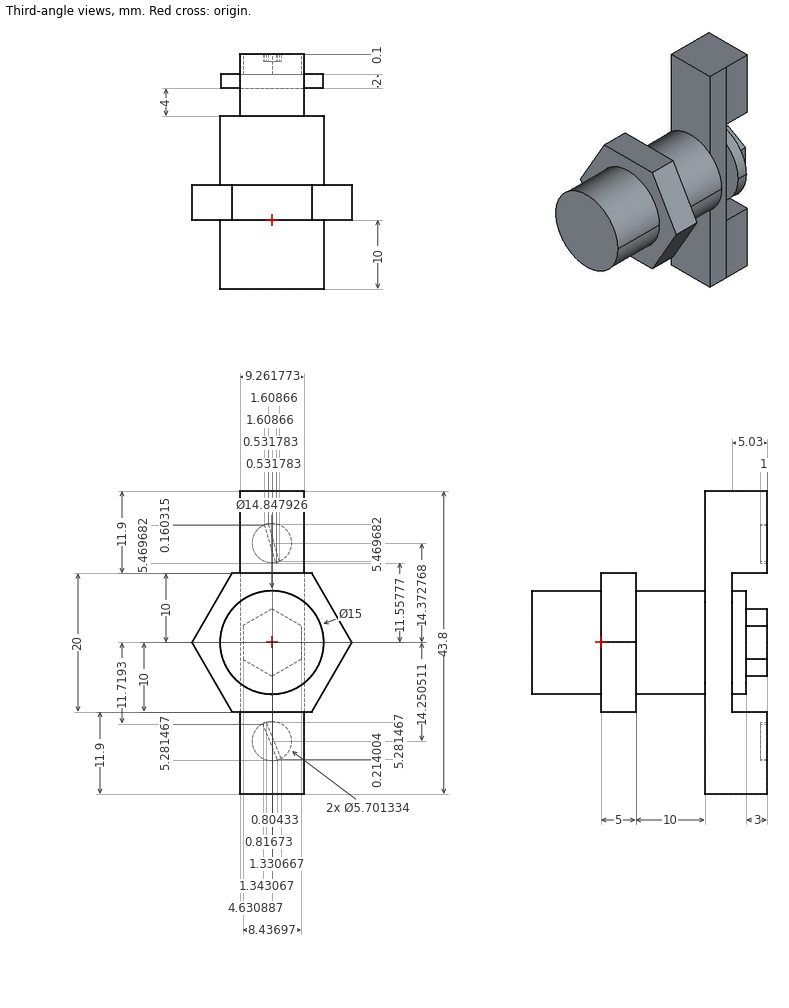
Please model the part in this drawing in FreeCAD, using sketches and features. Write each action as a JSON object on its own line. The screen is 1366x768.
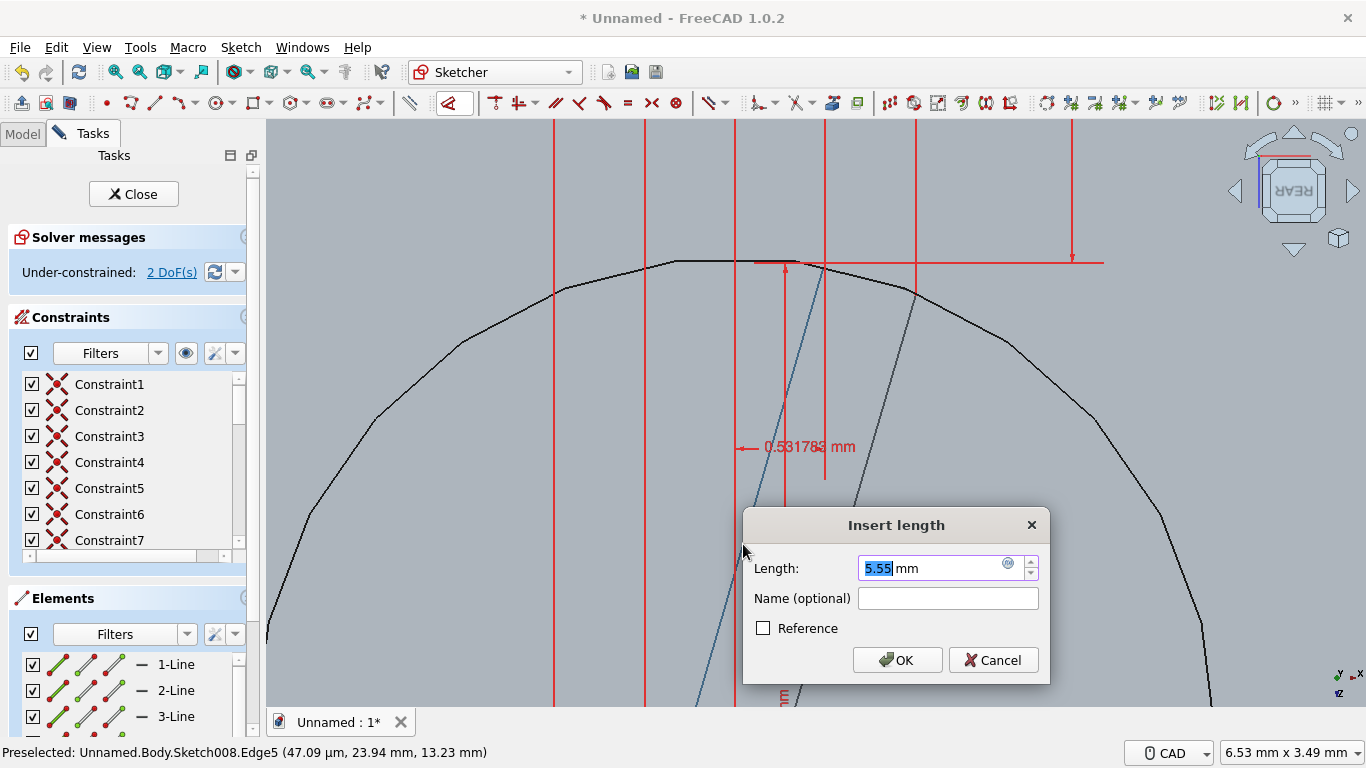
{"action": "type", "text": "5.469682"}
{"action": "key", "text": "Return"}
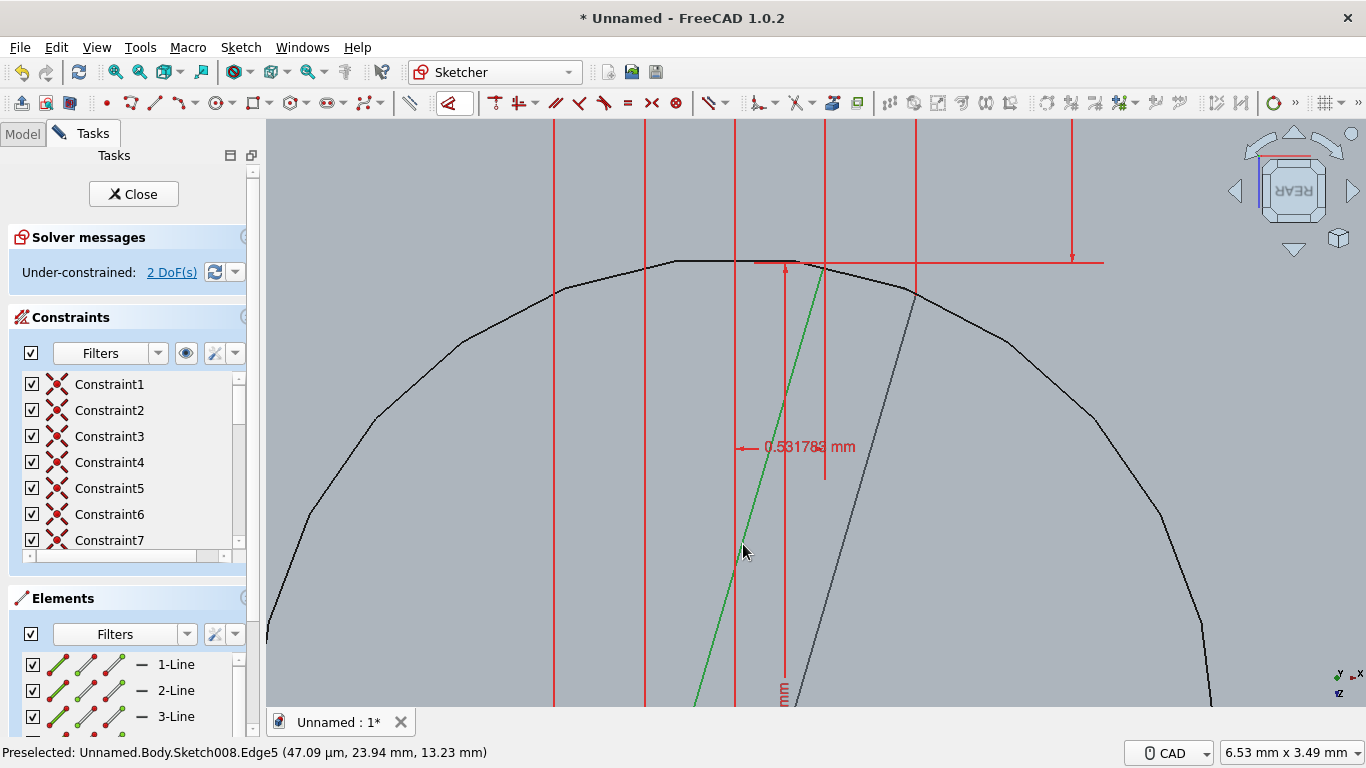
{"action": "scroll", "coordinate": [748, 548], "scroll_direction": "down", "scroll_amount": 14}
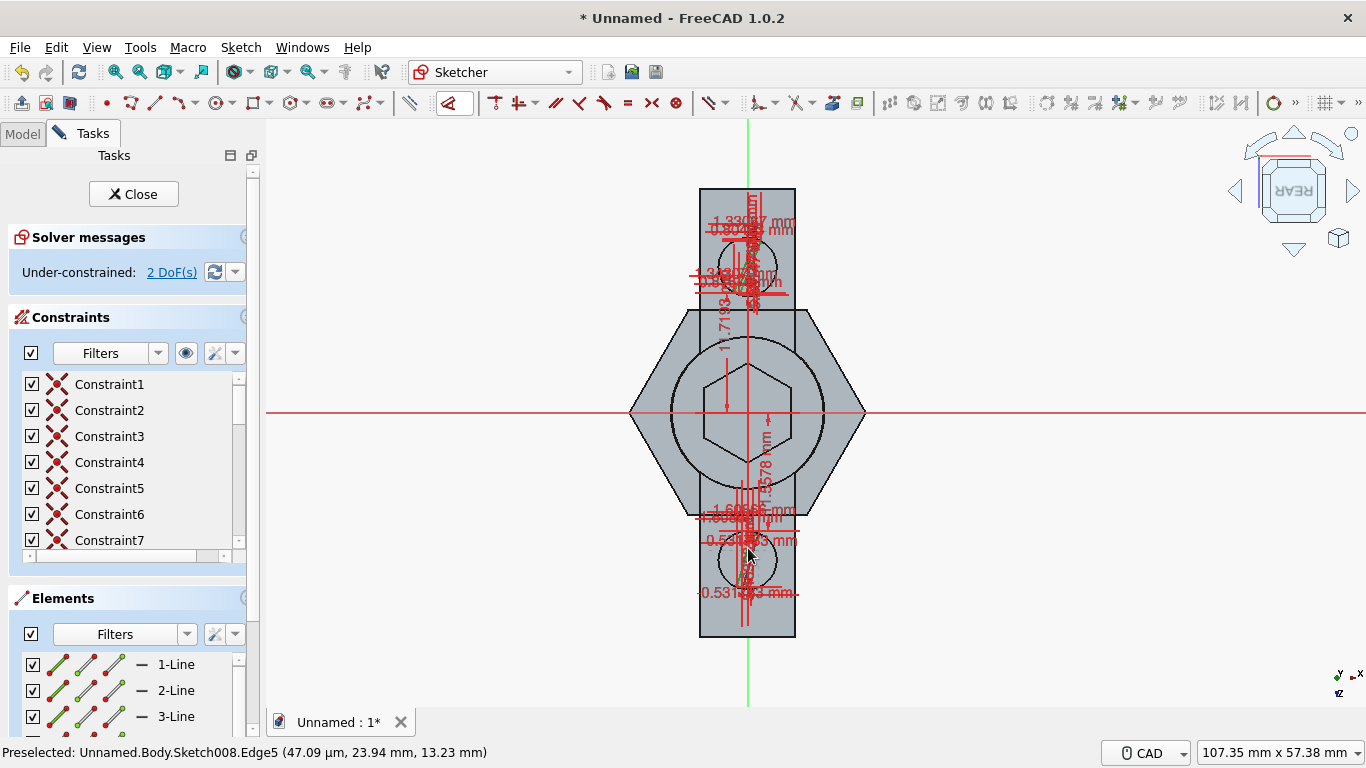
{"action": "scroll", "coordinate": [738, 588], "scroll_direction": "up", "scroll_amount": 16}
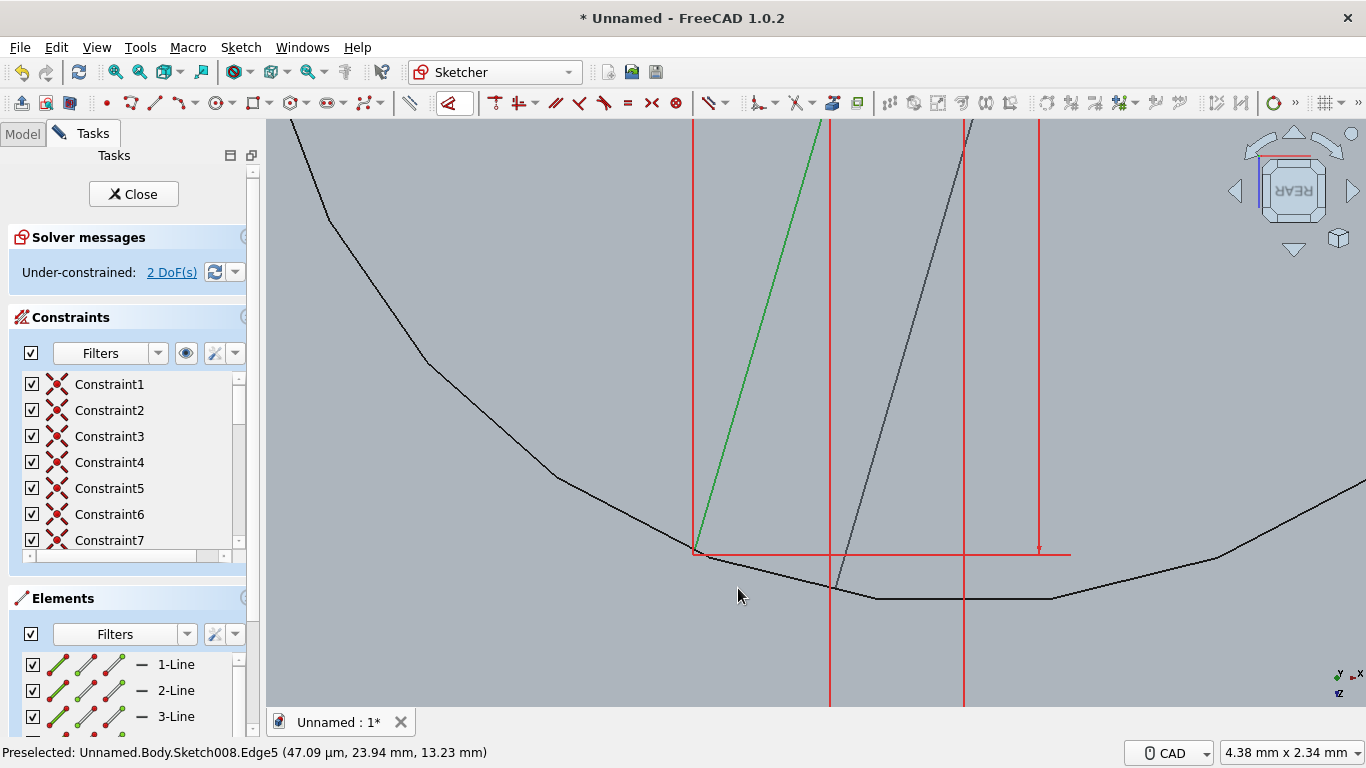
{"action": "left_click", "coordinate": [734, 570]}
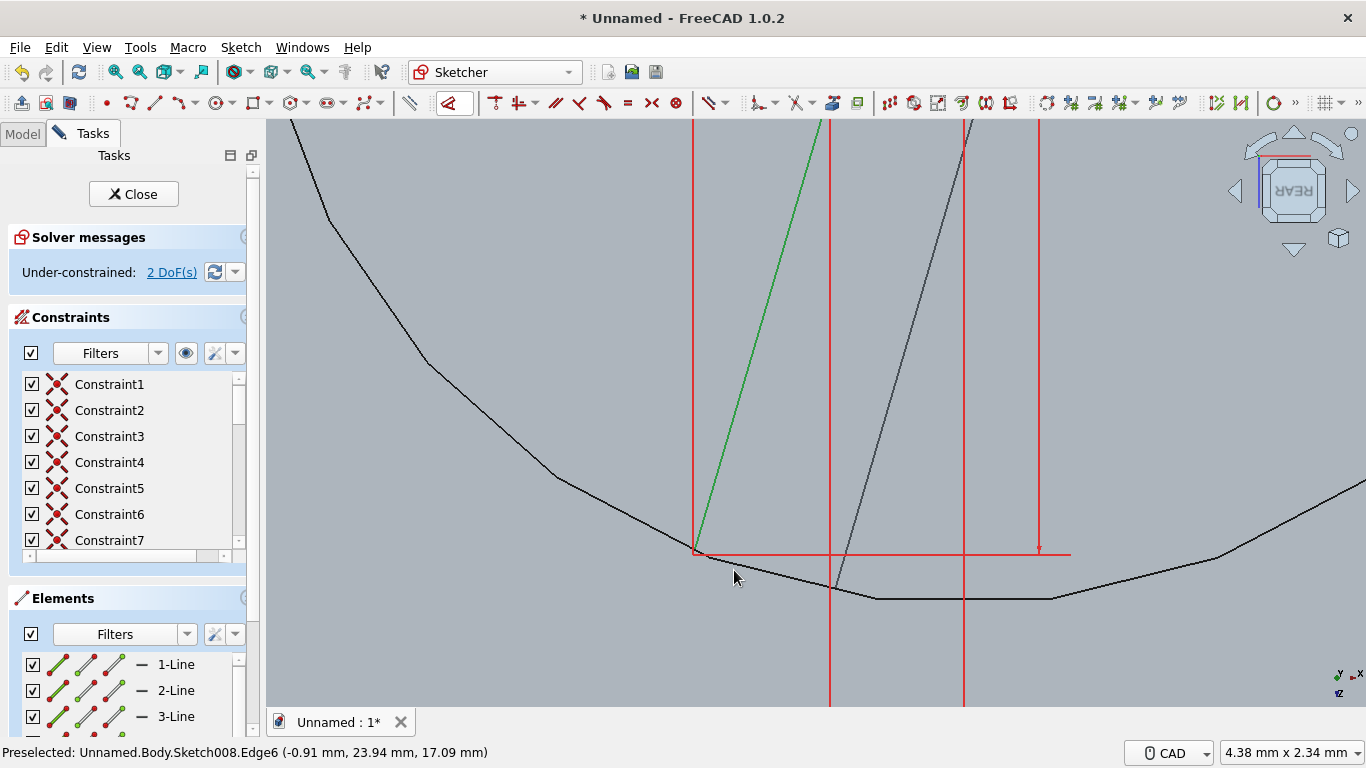
{"action": "left_click", "coordinate": [468, 104]}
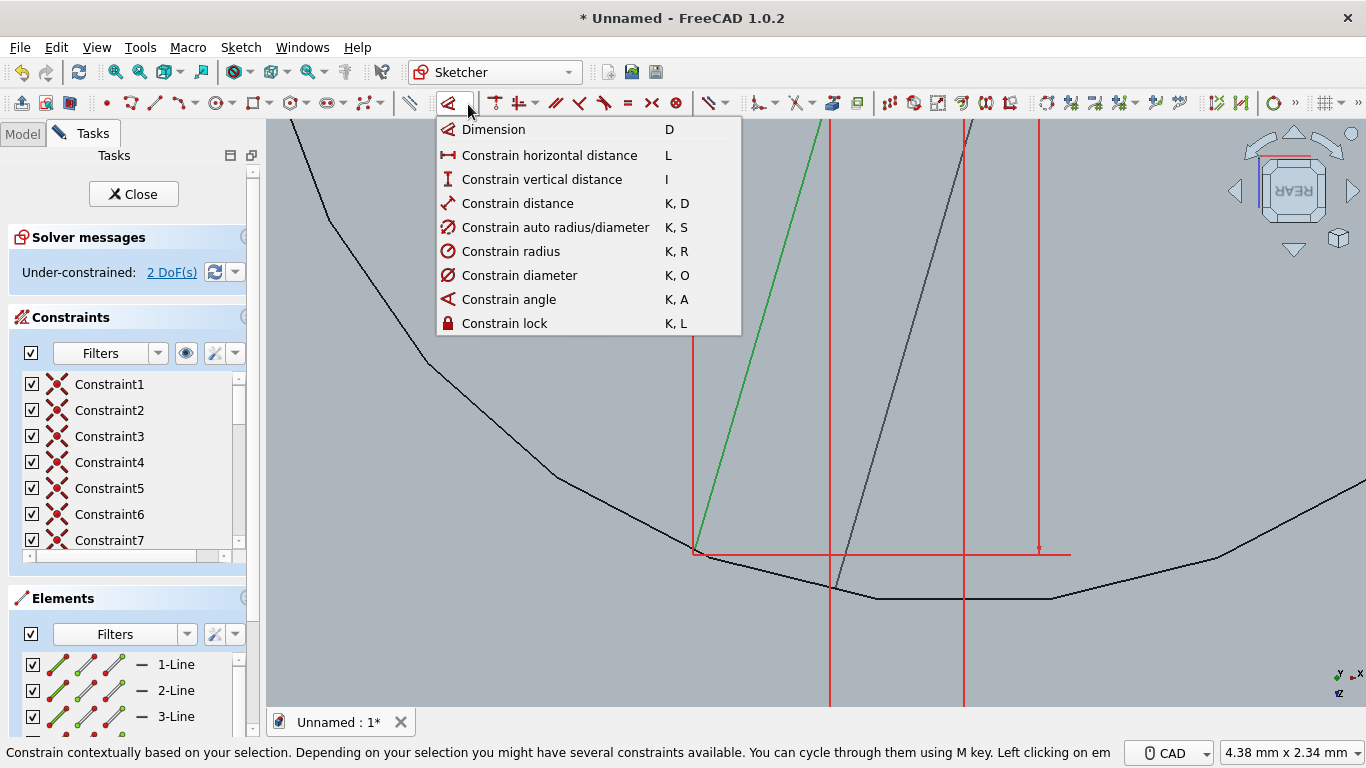
{"action": "left_click", "coordinate": [589, 179]}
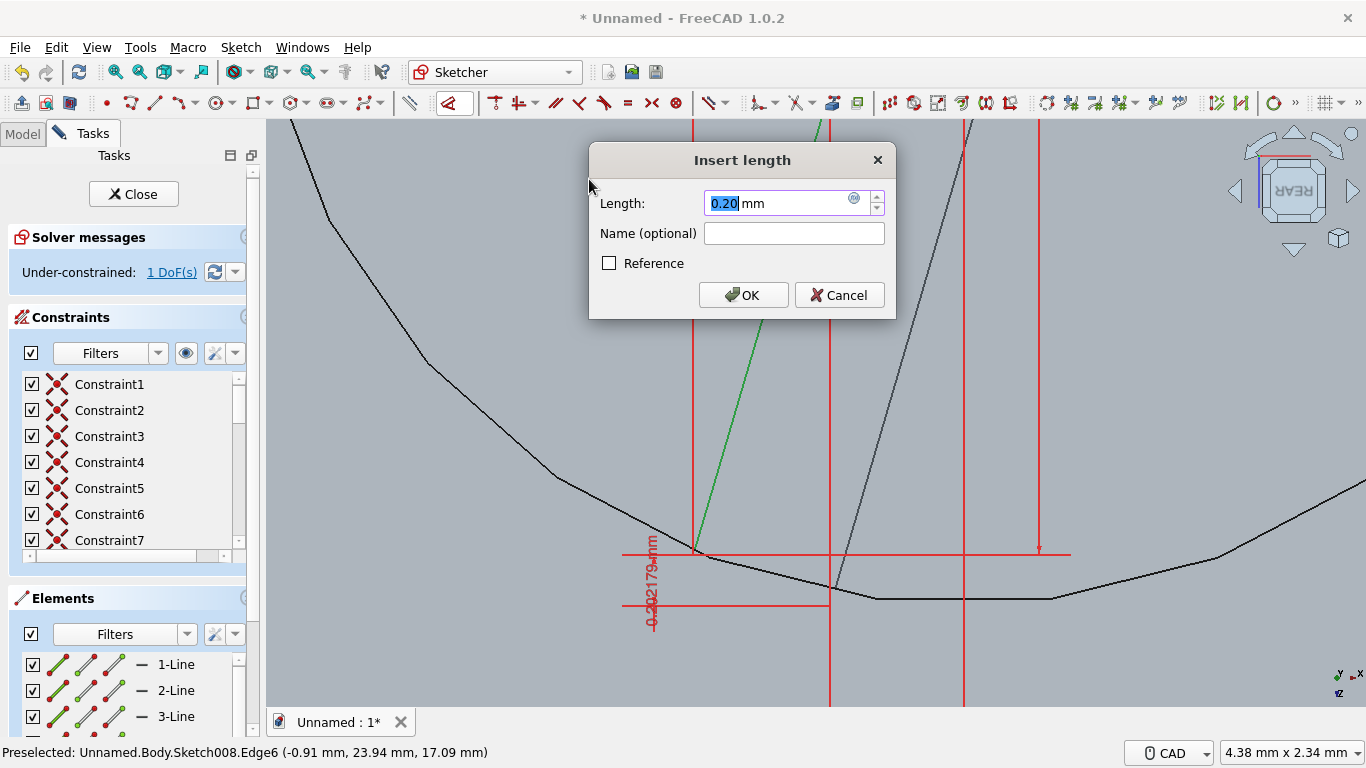
{"action": "type", "text": "0.160315"}
{"action": "key", "text": "Return"}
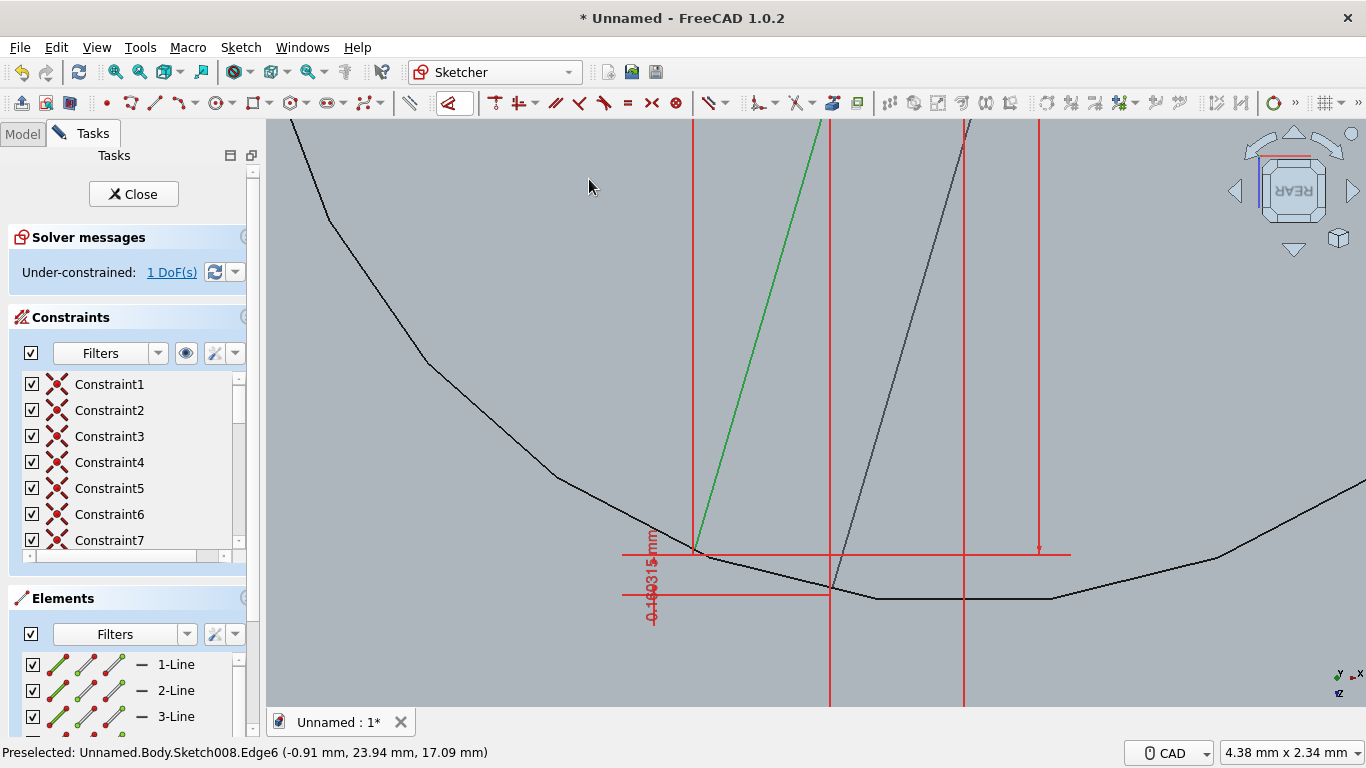
{"action": "left_click", "coordinate": [952, 184]}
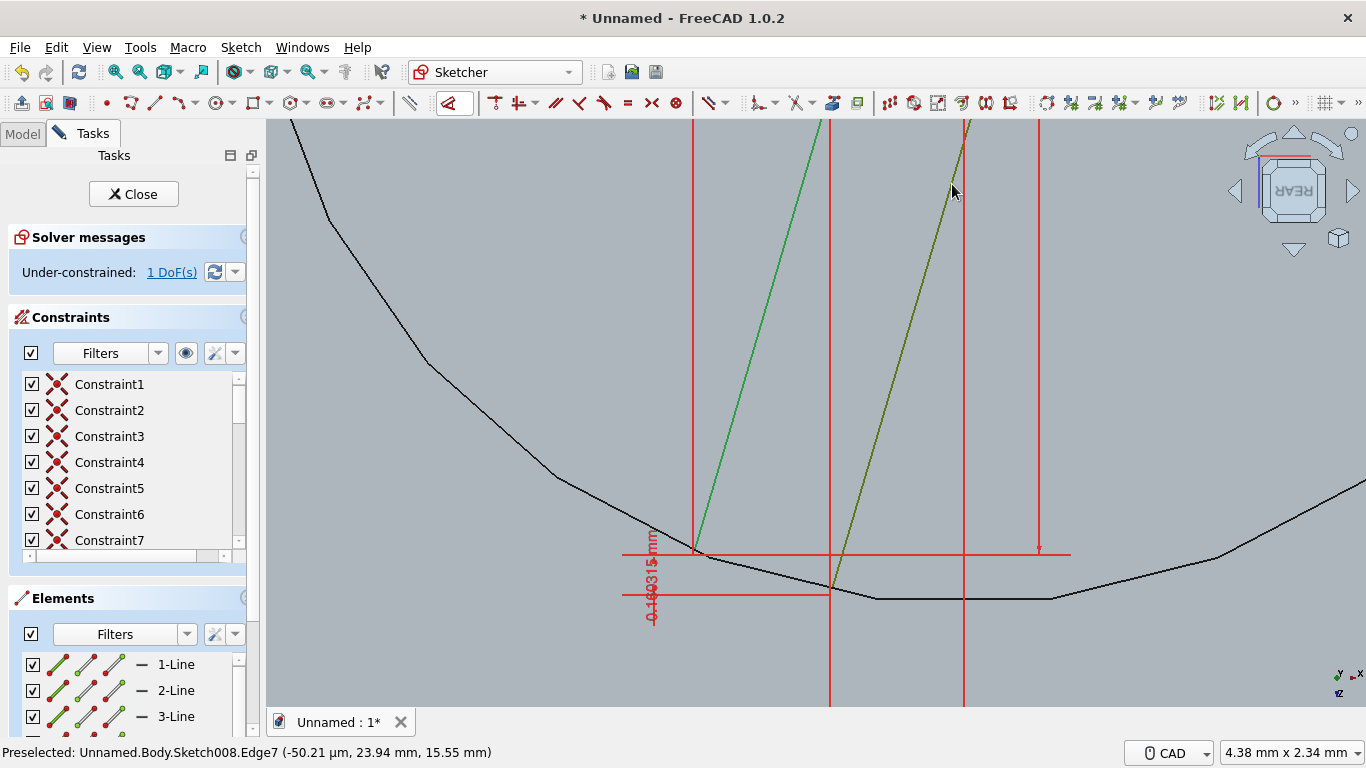
{"action": "left_click", "coordinate": [468, 104]}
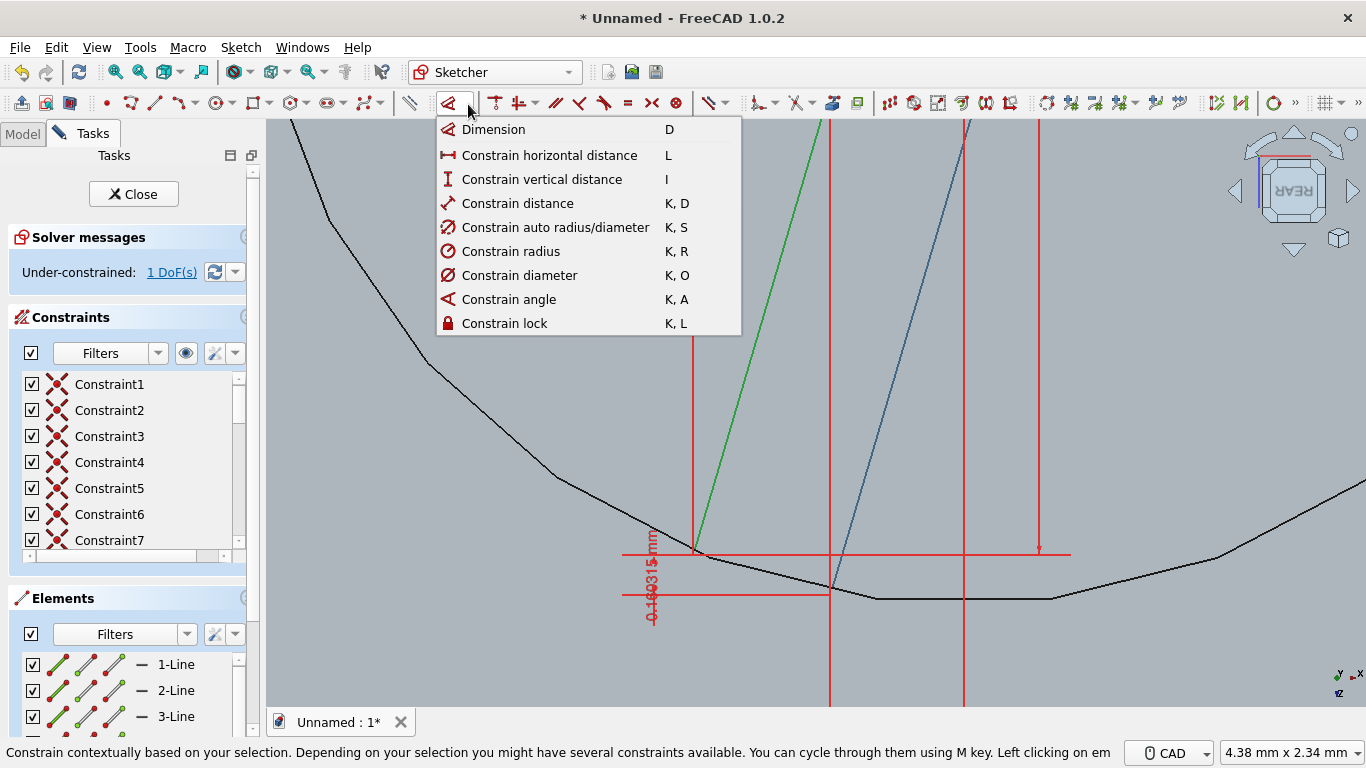
{"action": "left_click", "coordinate": [589, 179]}